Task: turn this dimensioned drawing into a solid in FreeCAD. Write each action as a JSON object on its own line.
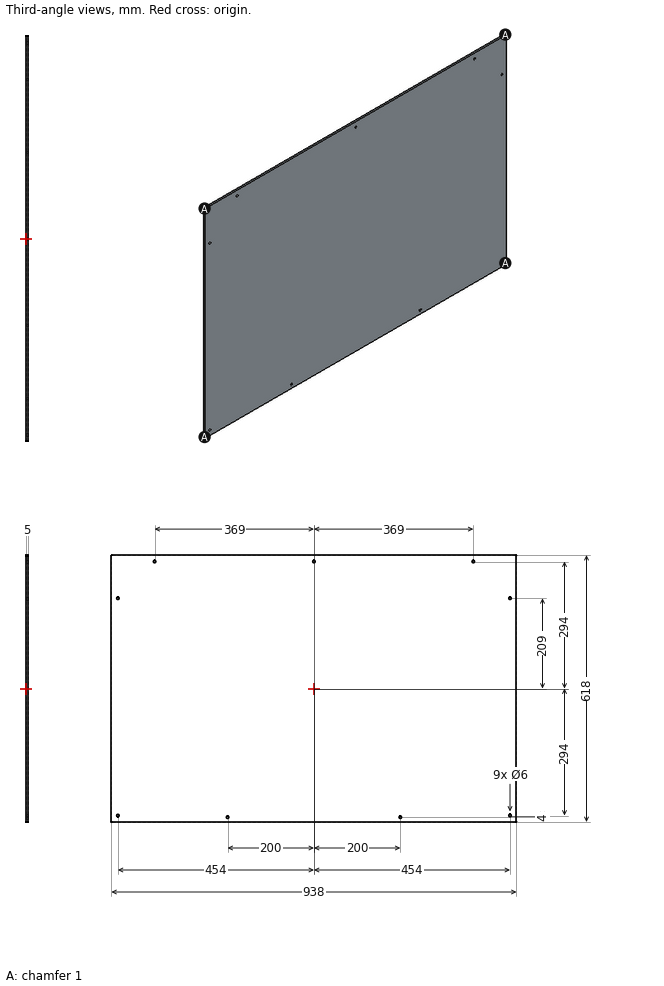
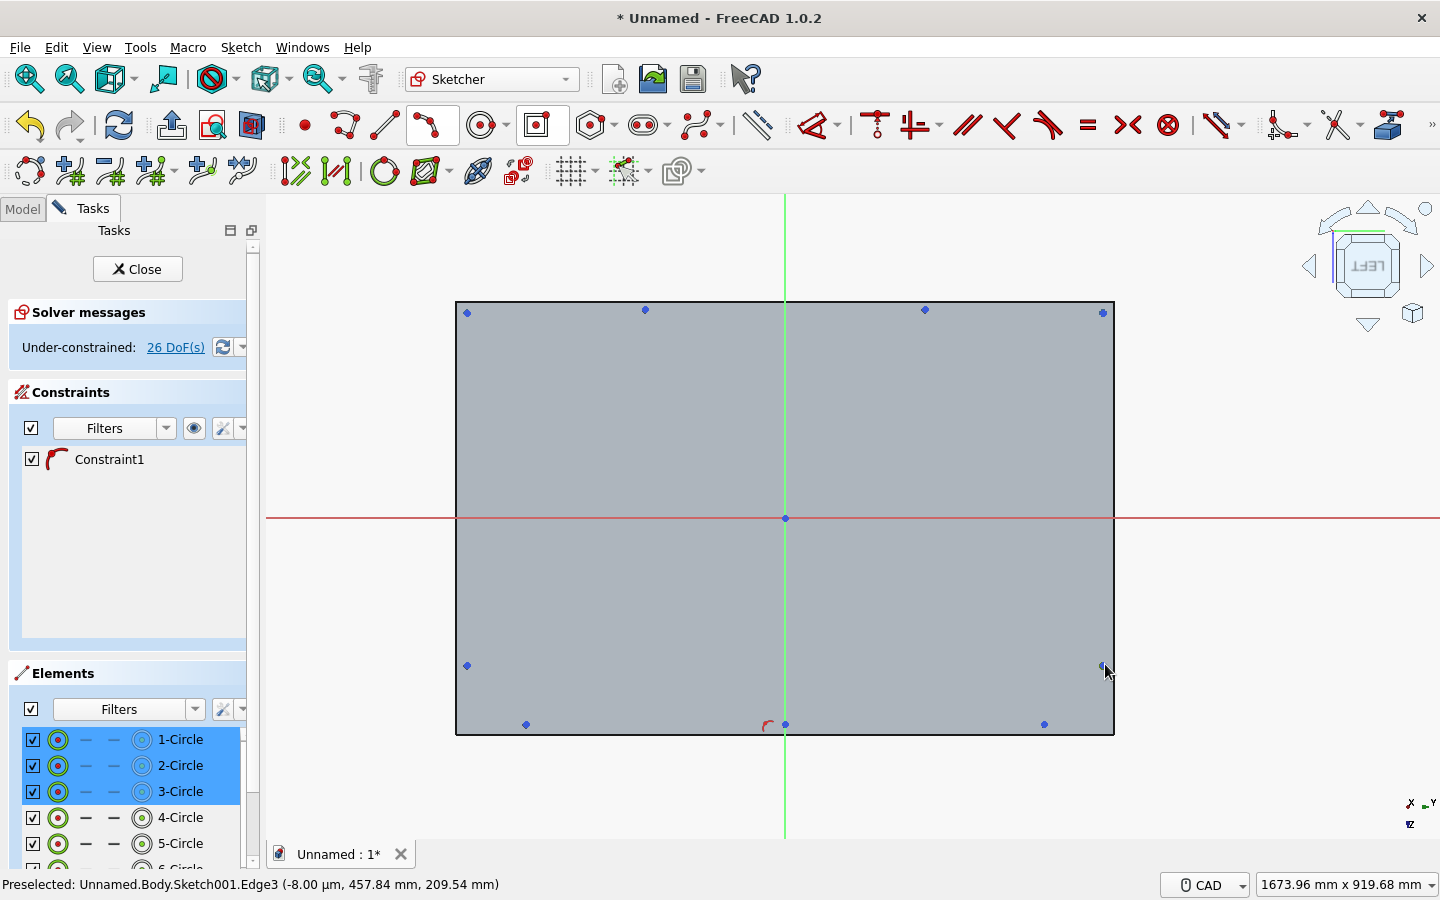
{"action": "scroll", "coordinate": [1046, 723], "scroll_direction": "up", "scroll_amount": 9}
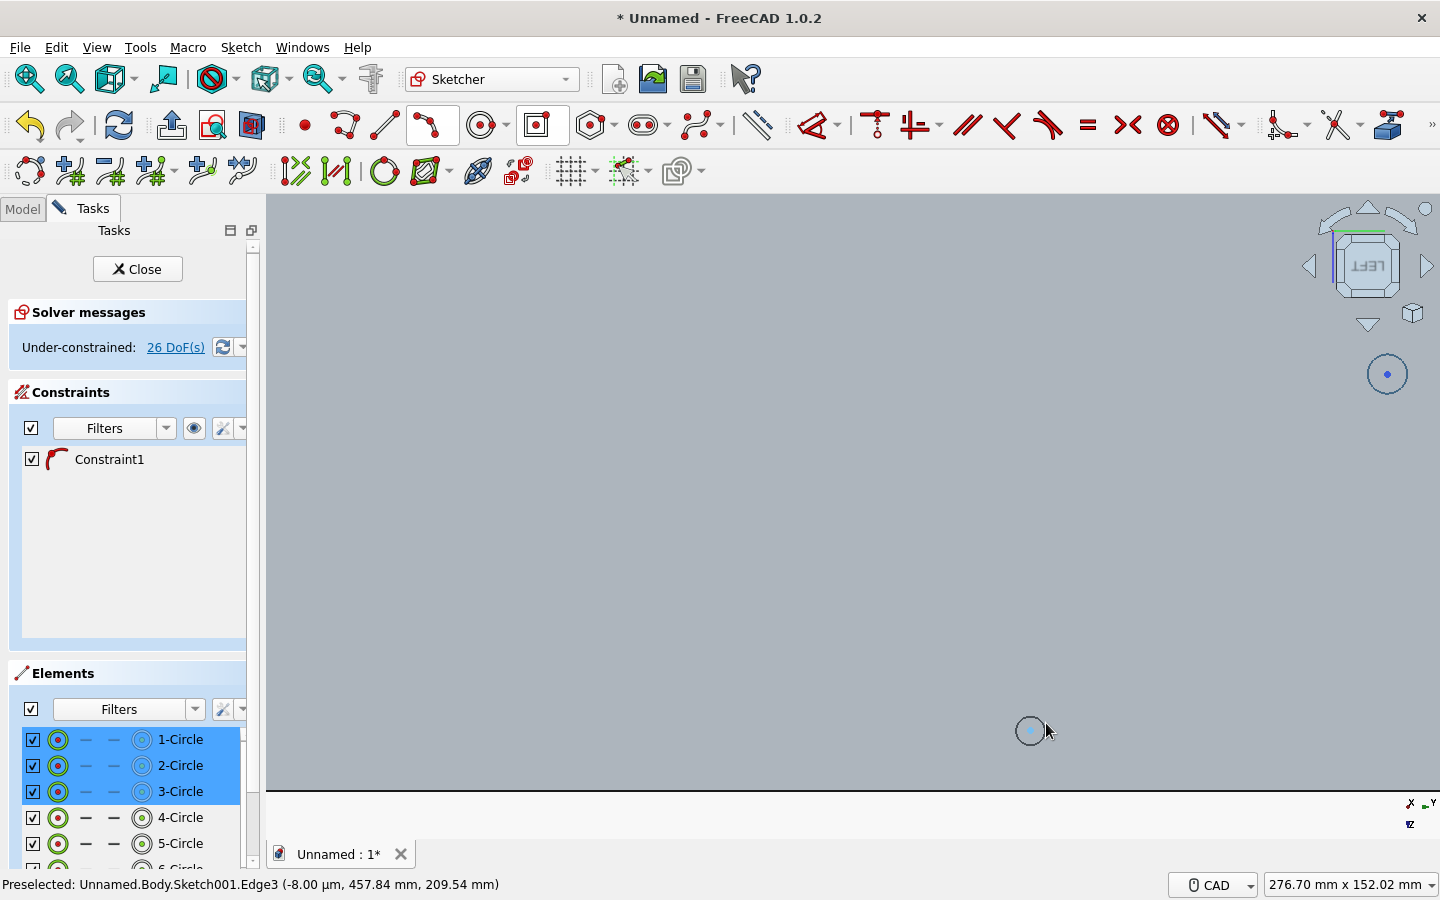
{"action": "left_click", "coordinate": [1041, 721]}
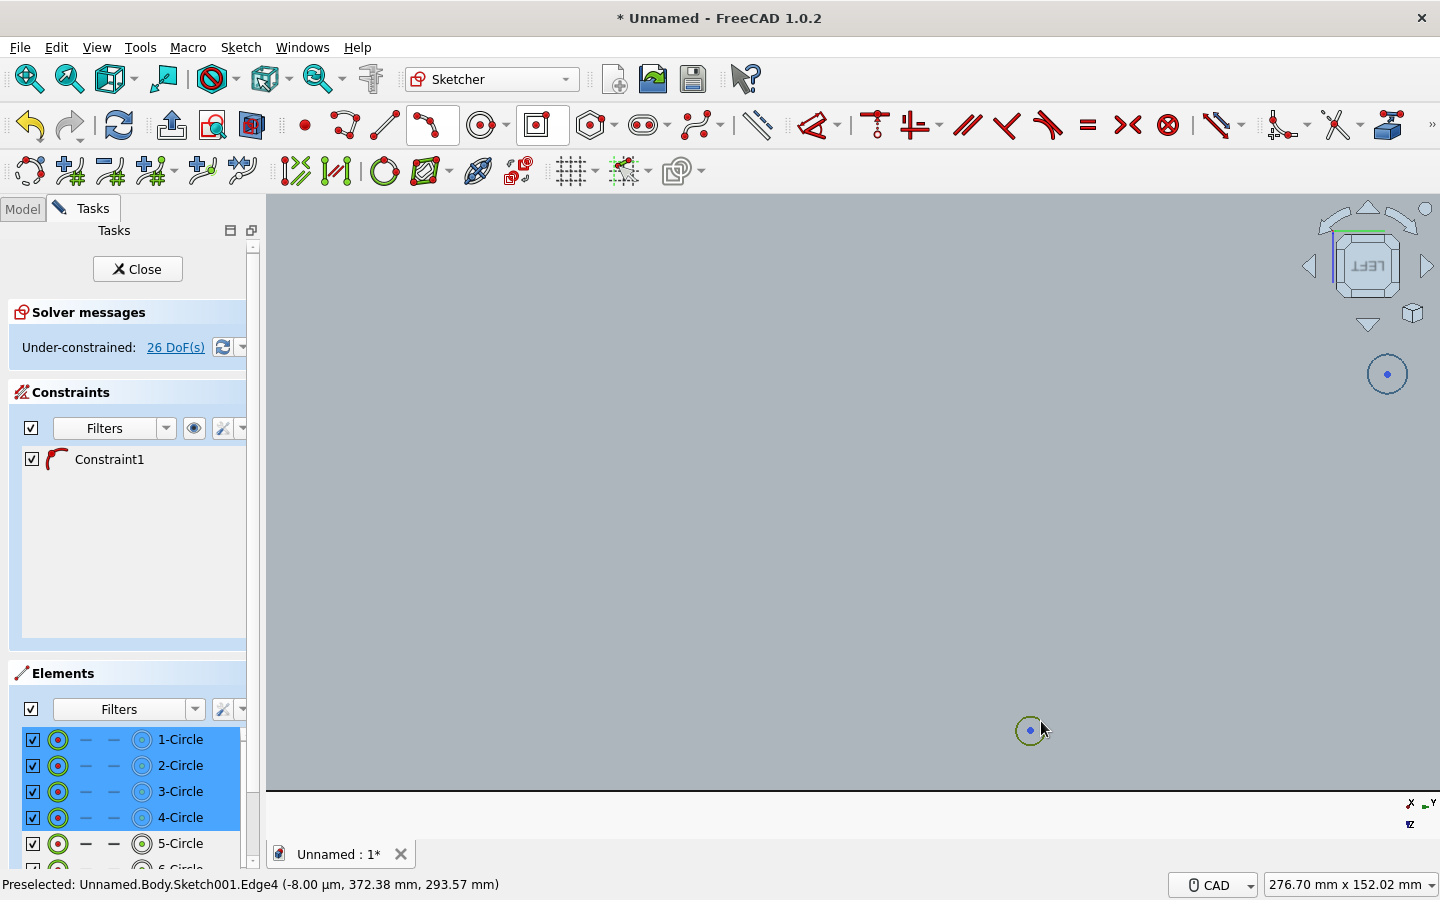
{"action": "scroll", "coordinate": [1046, 723], "scroll_direction": "down", "scroll_amount": 9}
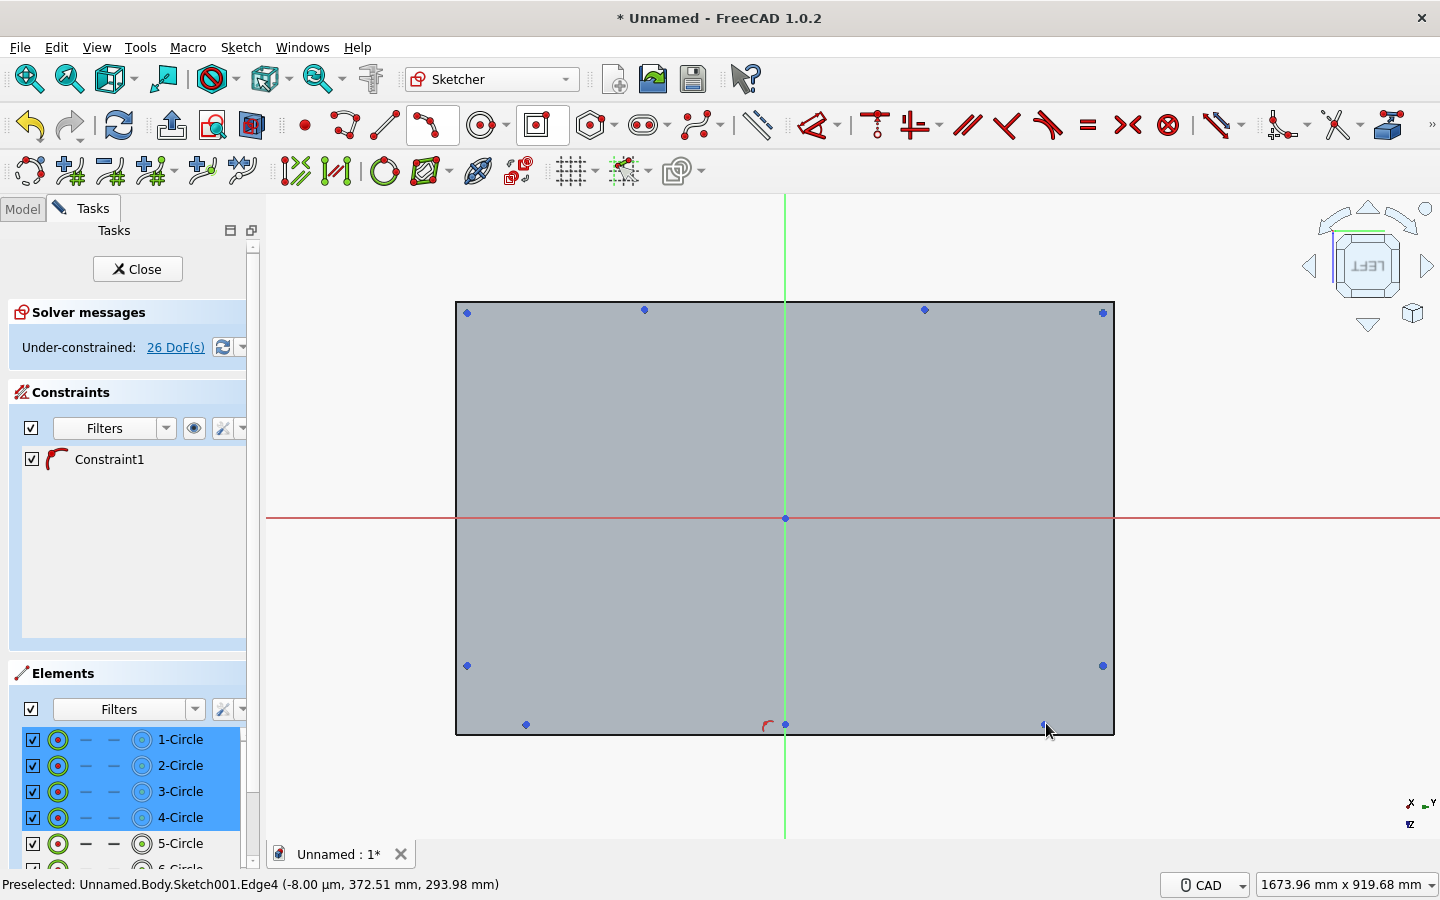
{"action": "scroll", "coordinate": [528, 723], "scroll_direction": "up", "scroll_amount": 9}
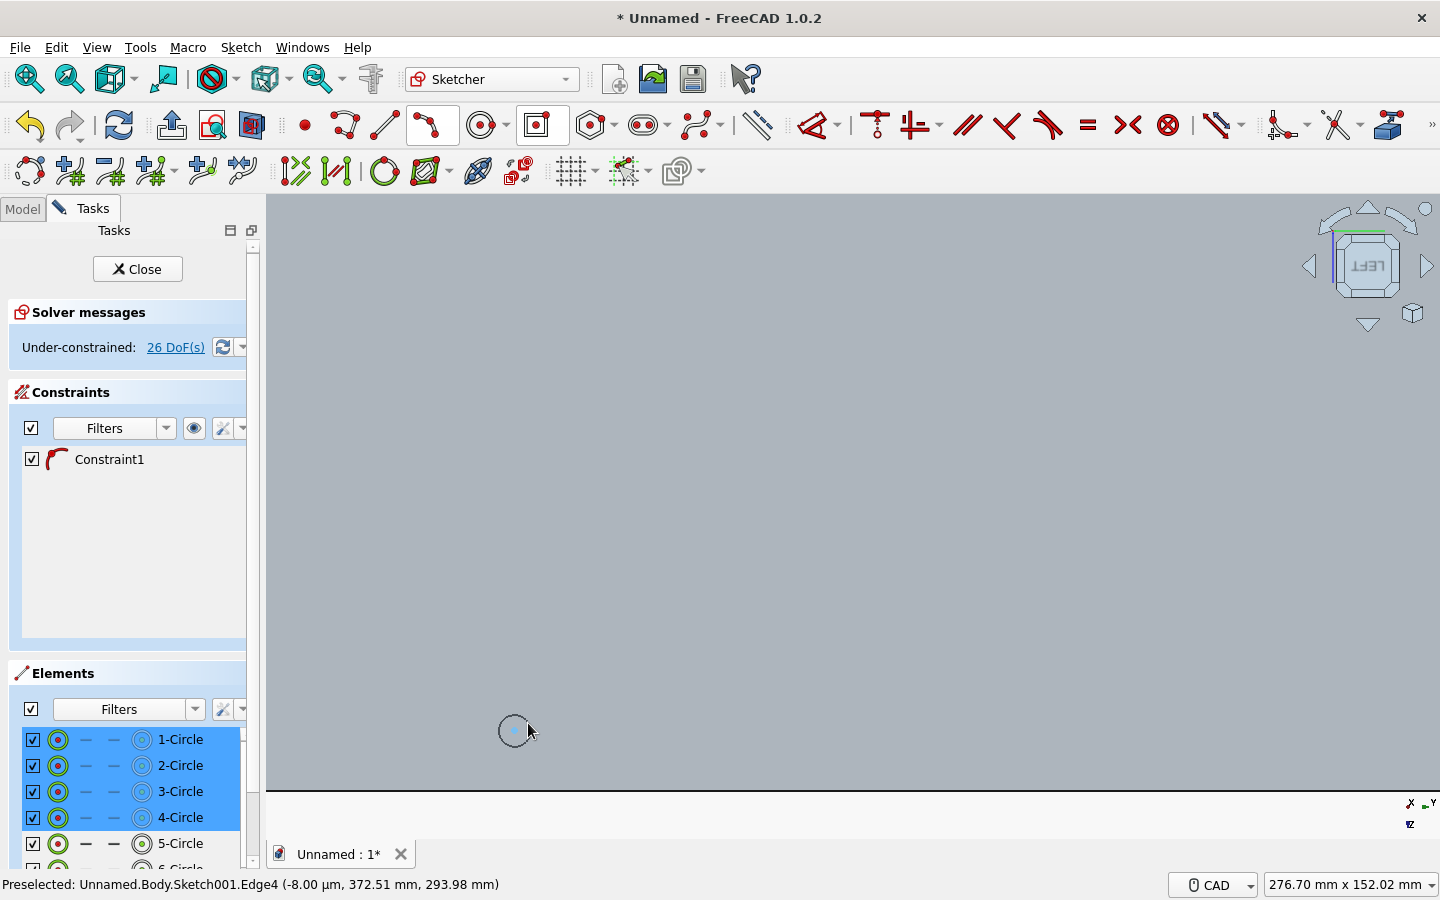
{"action": "left_click", "coordinate": [526, 720]}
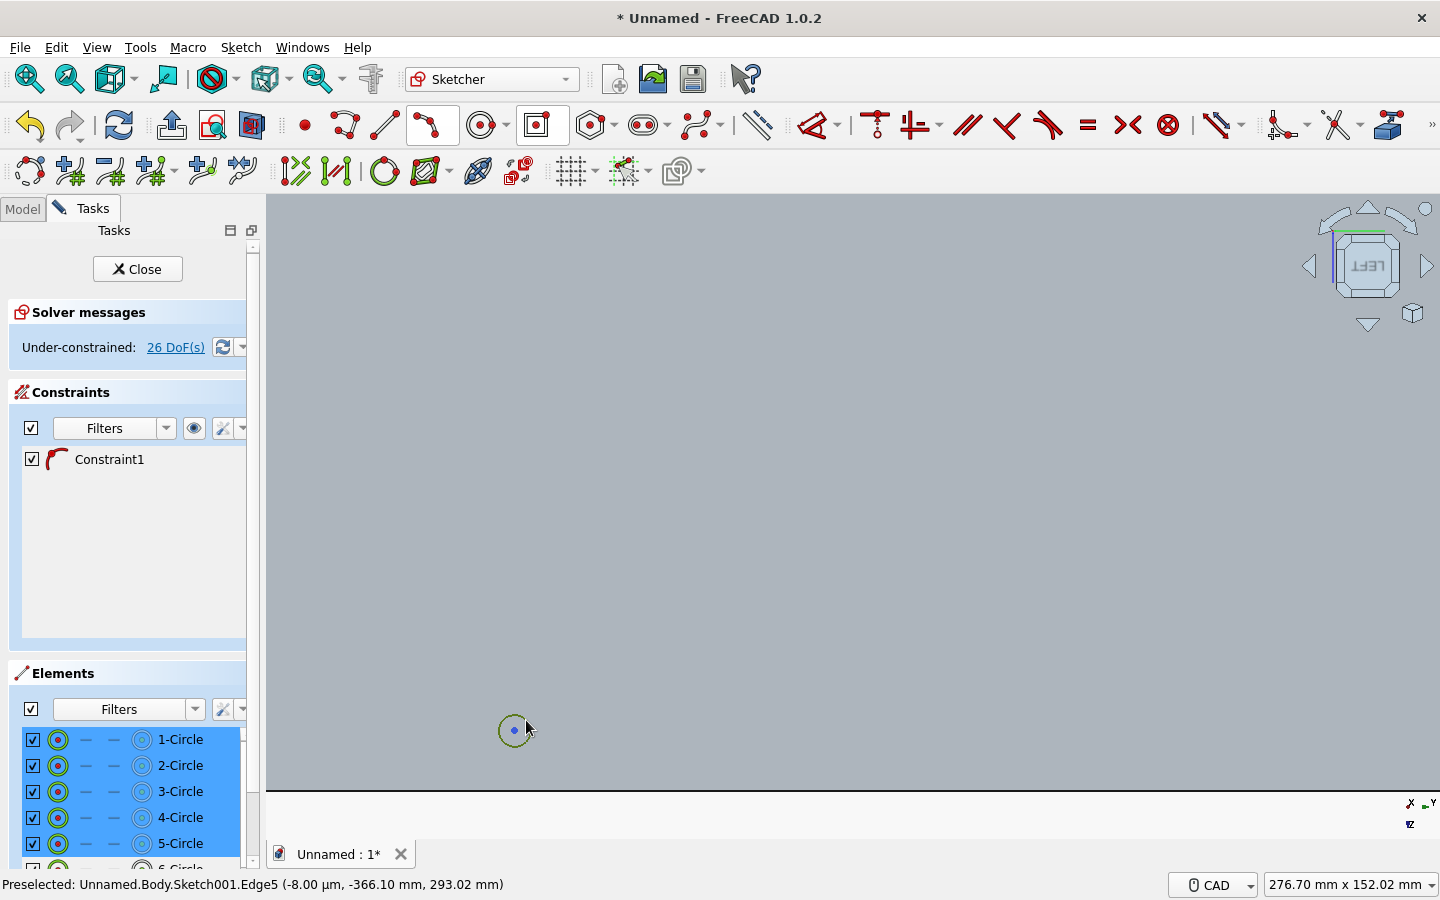
{"action": "scroll", "coordinate": [528, 723], "scroll_direction": "down", "scroll_amount": 9}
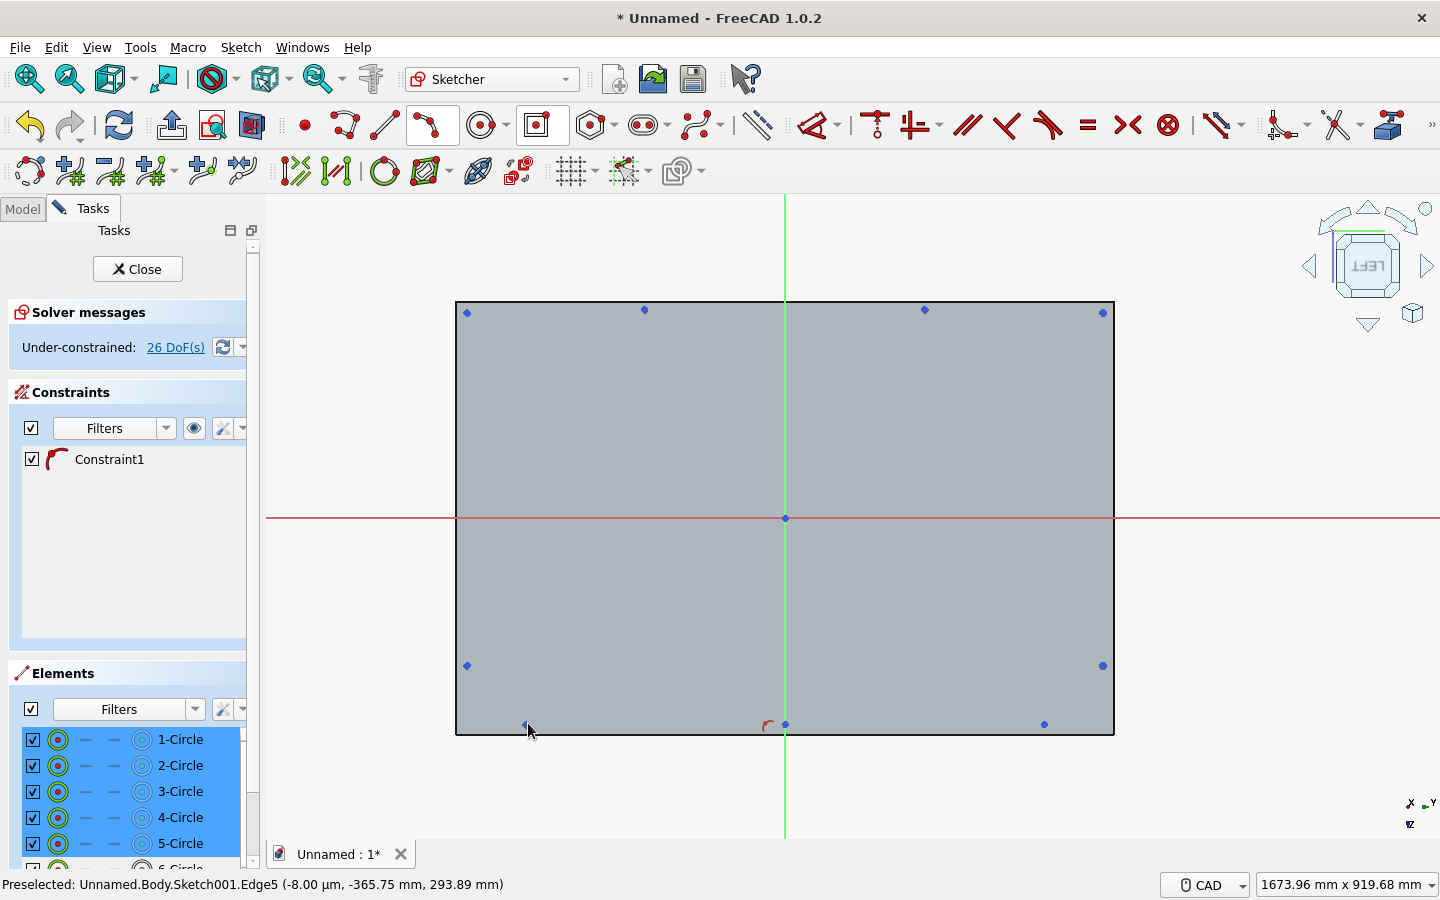
{"action": "scroll", "coordinate": [469, 664], "scroll_direction": "up", "scroll_amount": 8}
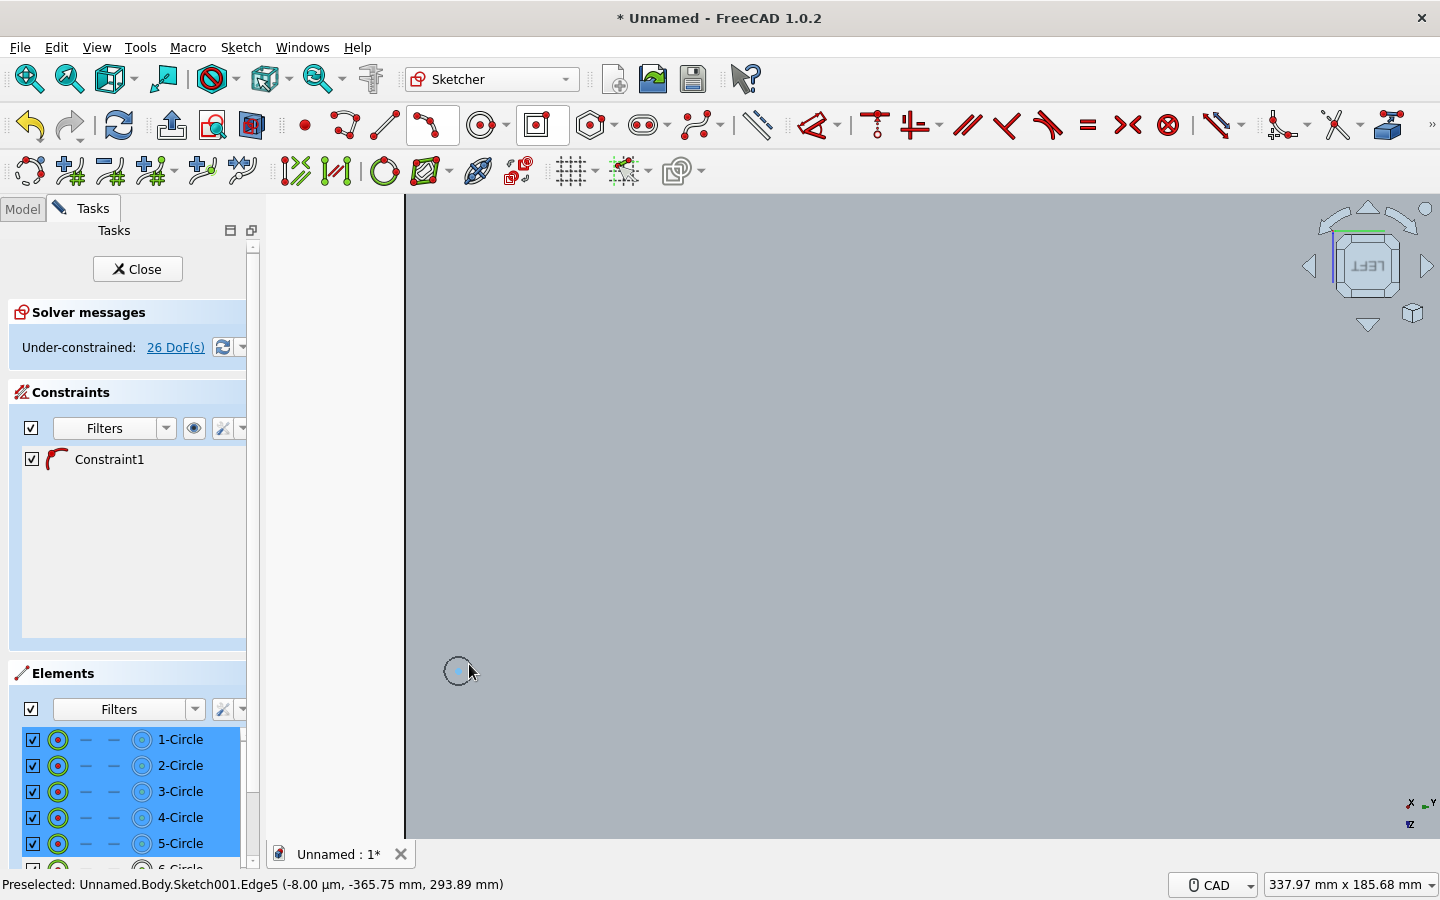
{"action": "left_click", "coordinate": [468, 661]}